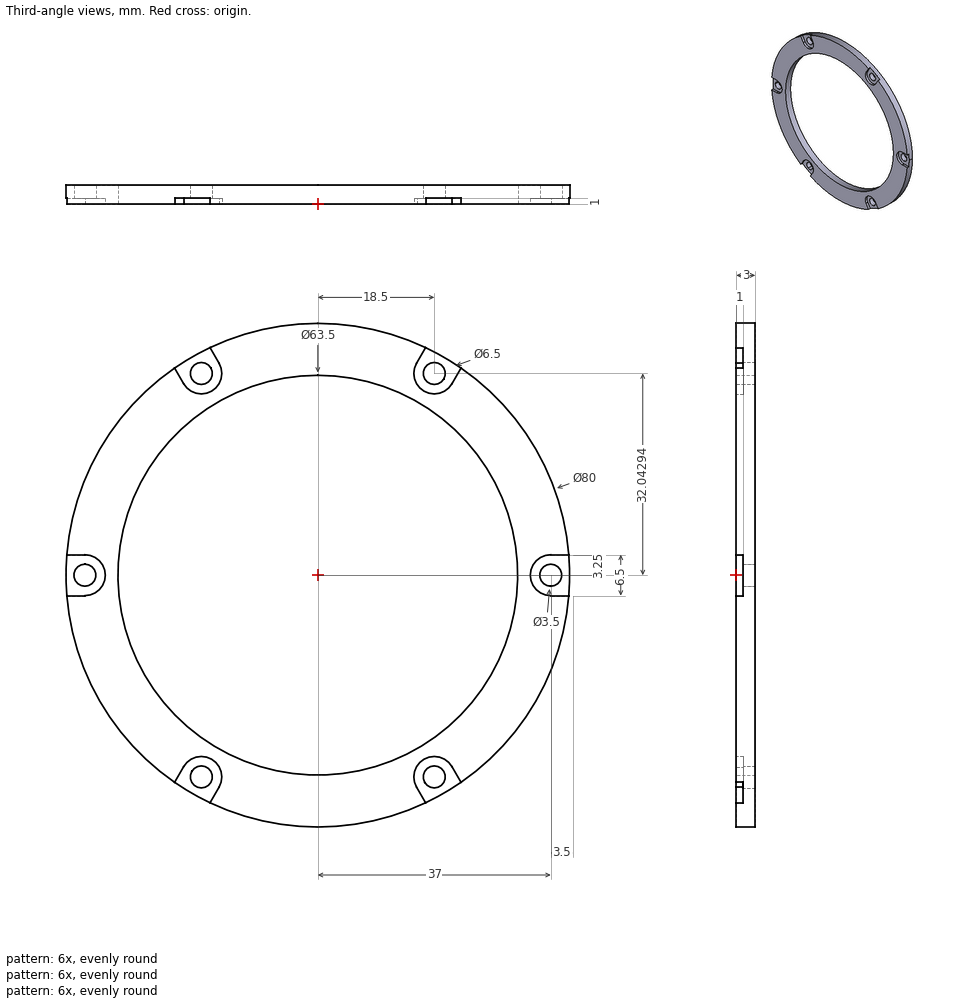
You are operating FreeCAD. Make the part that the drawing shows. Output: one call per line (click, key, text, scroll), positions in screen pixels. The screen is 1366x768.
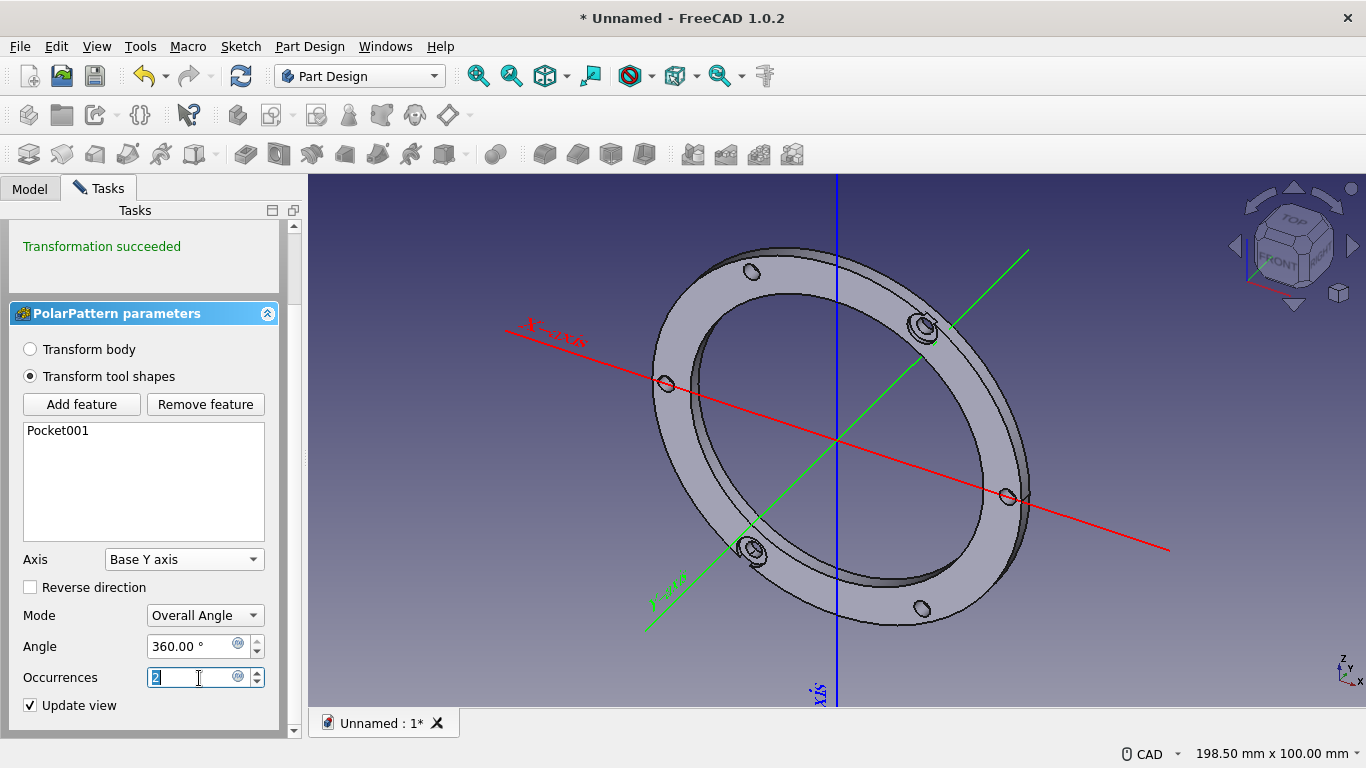
text(6)
key(Tab)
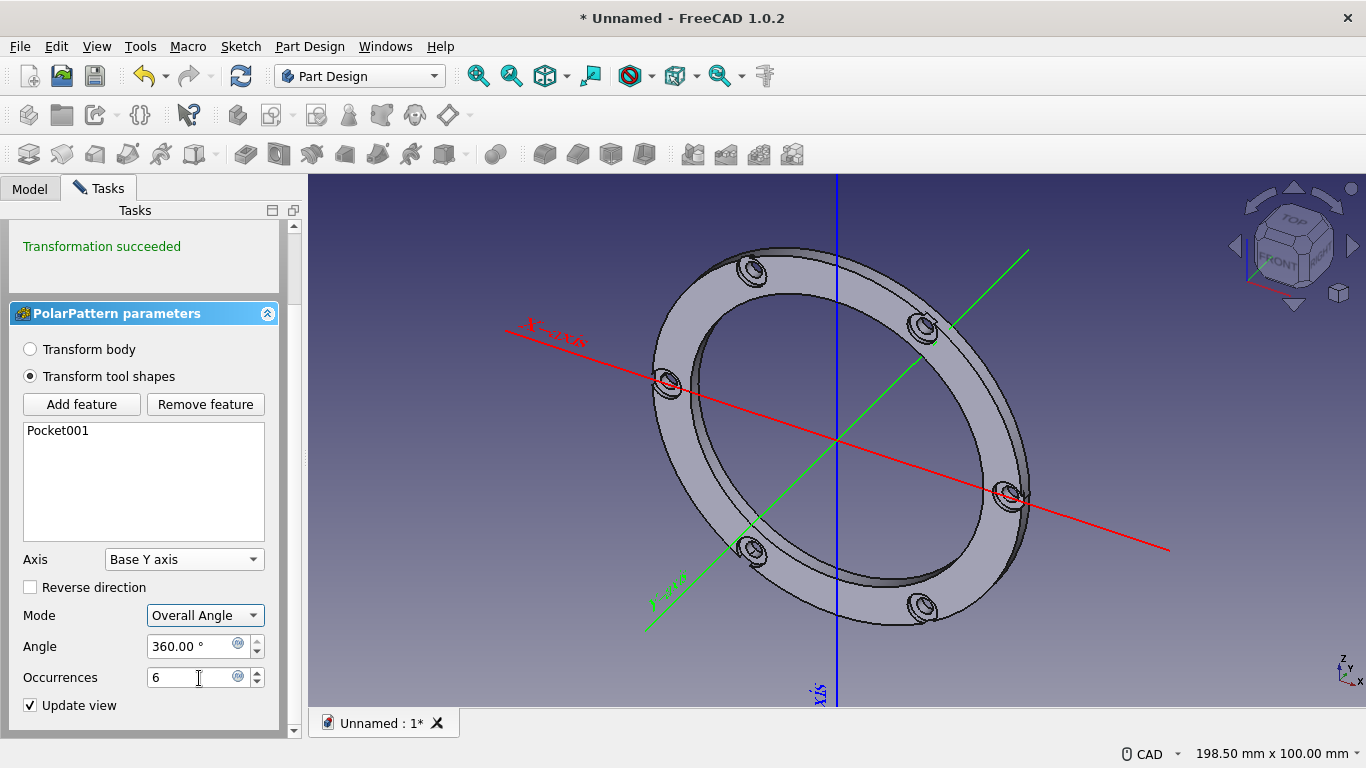
scroll(294, 479, up, 3)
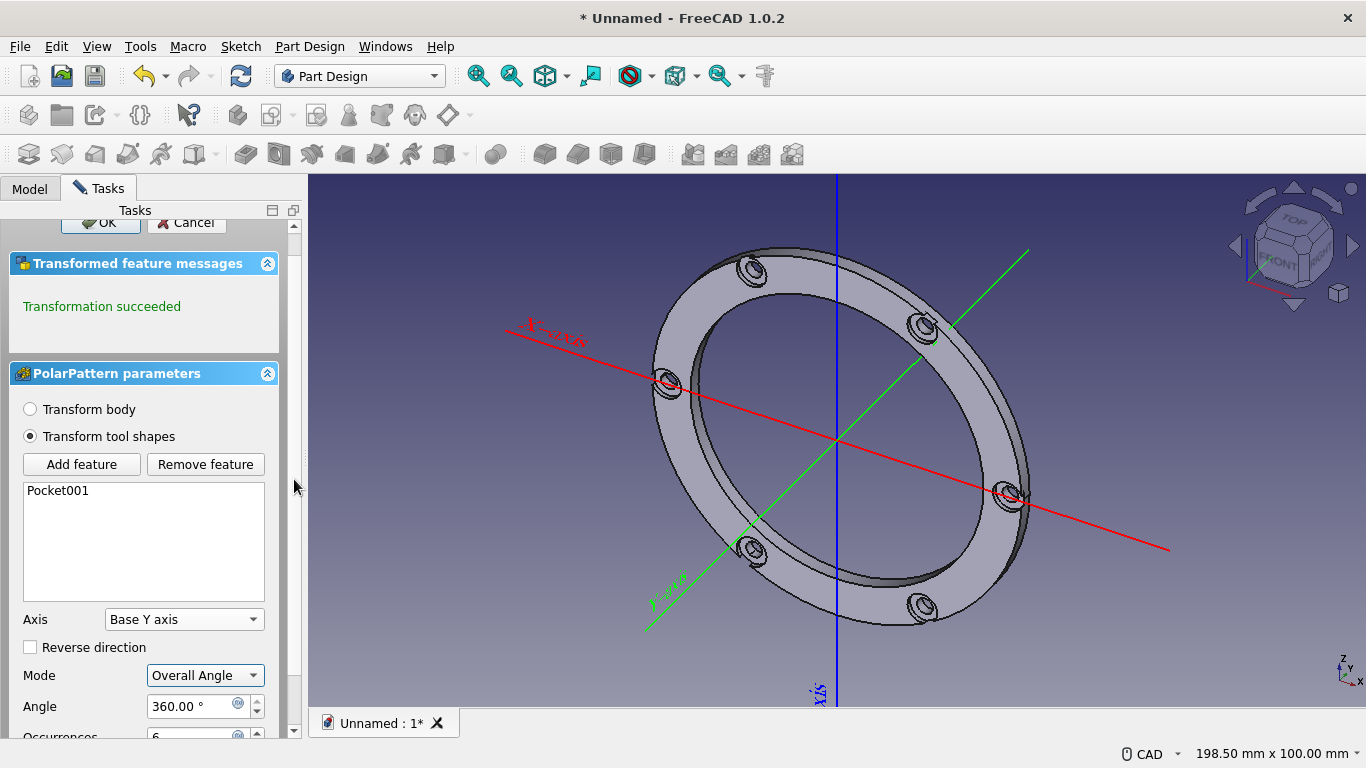
click(101, 249)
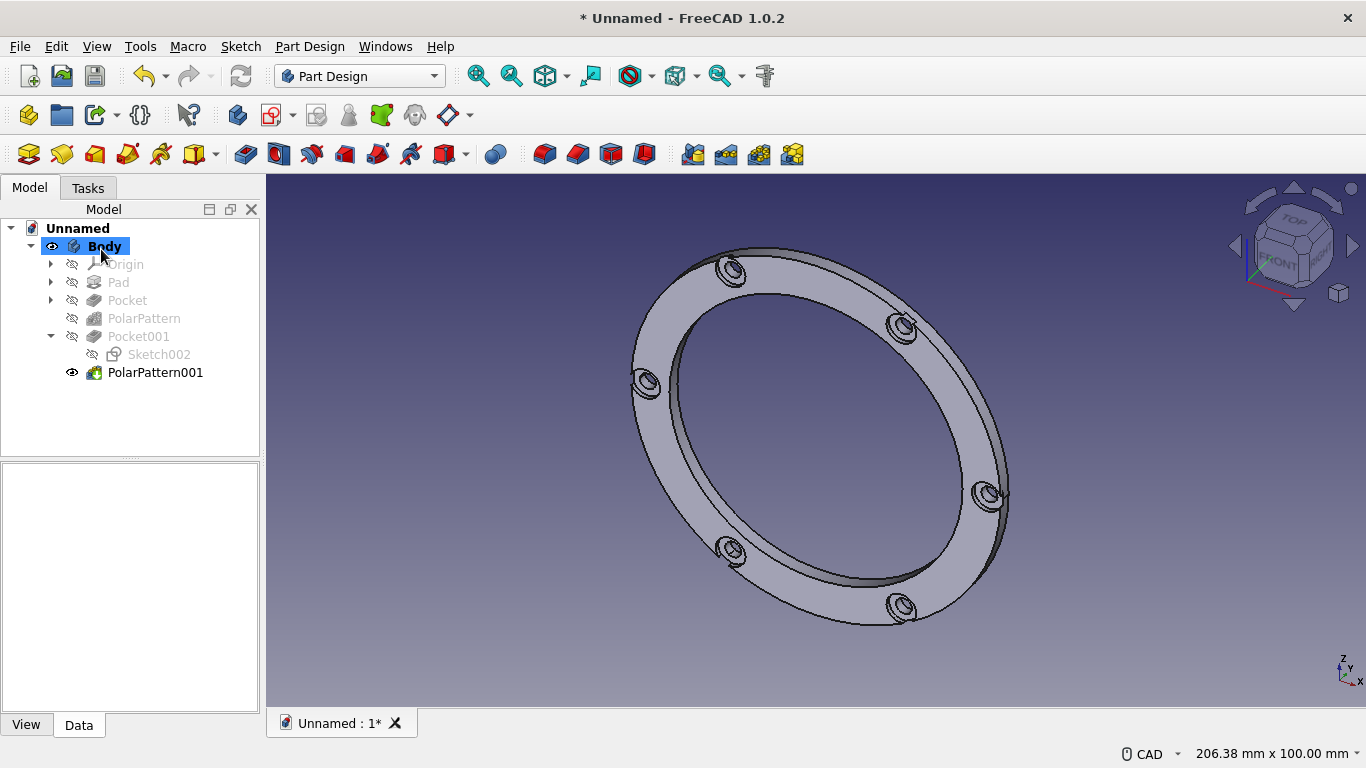
click(974, 542)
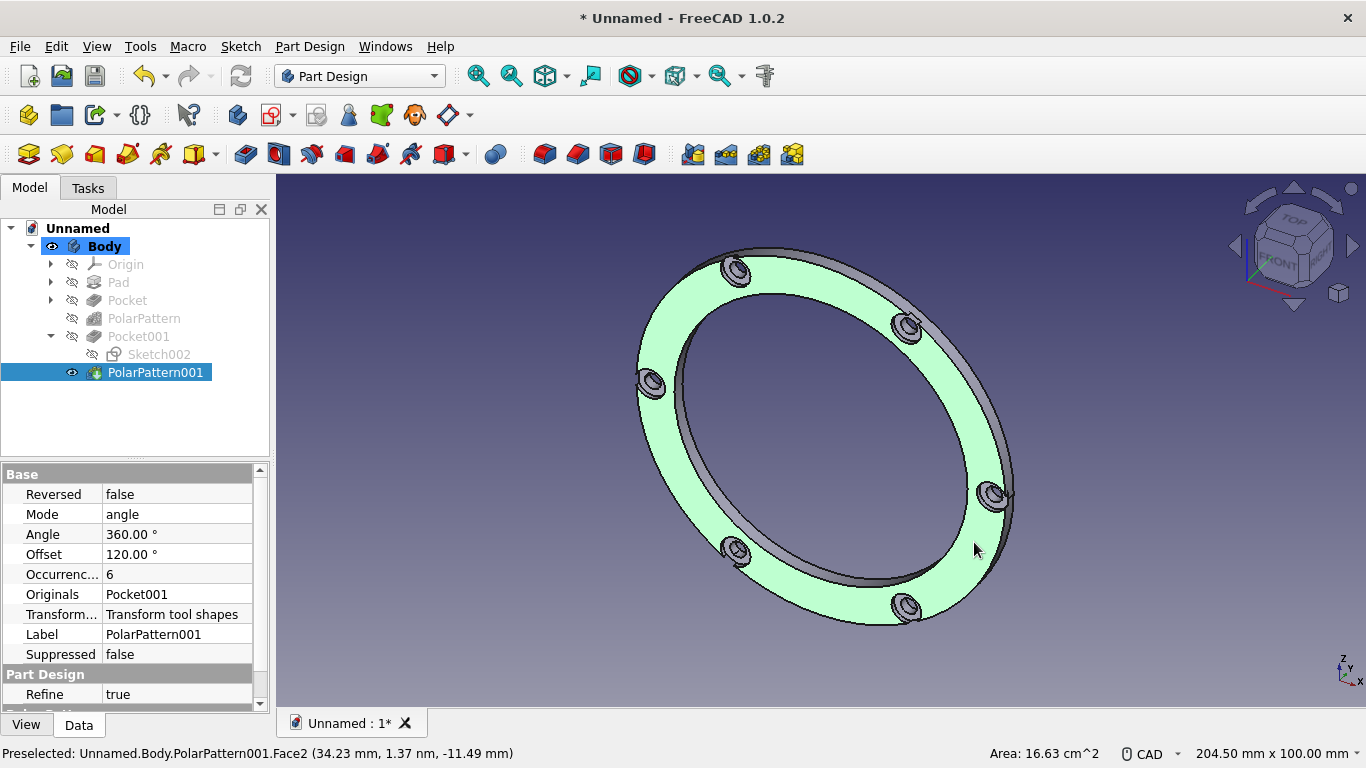
click(270, 116)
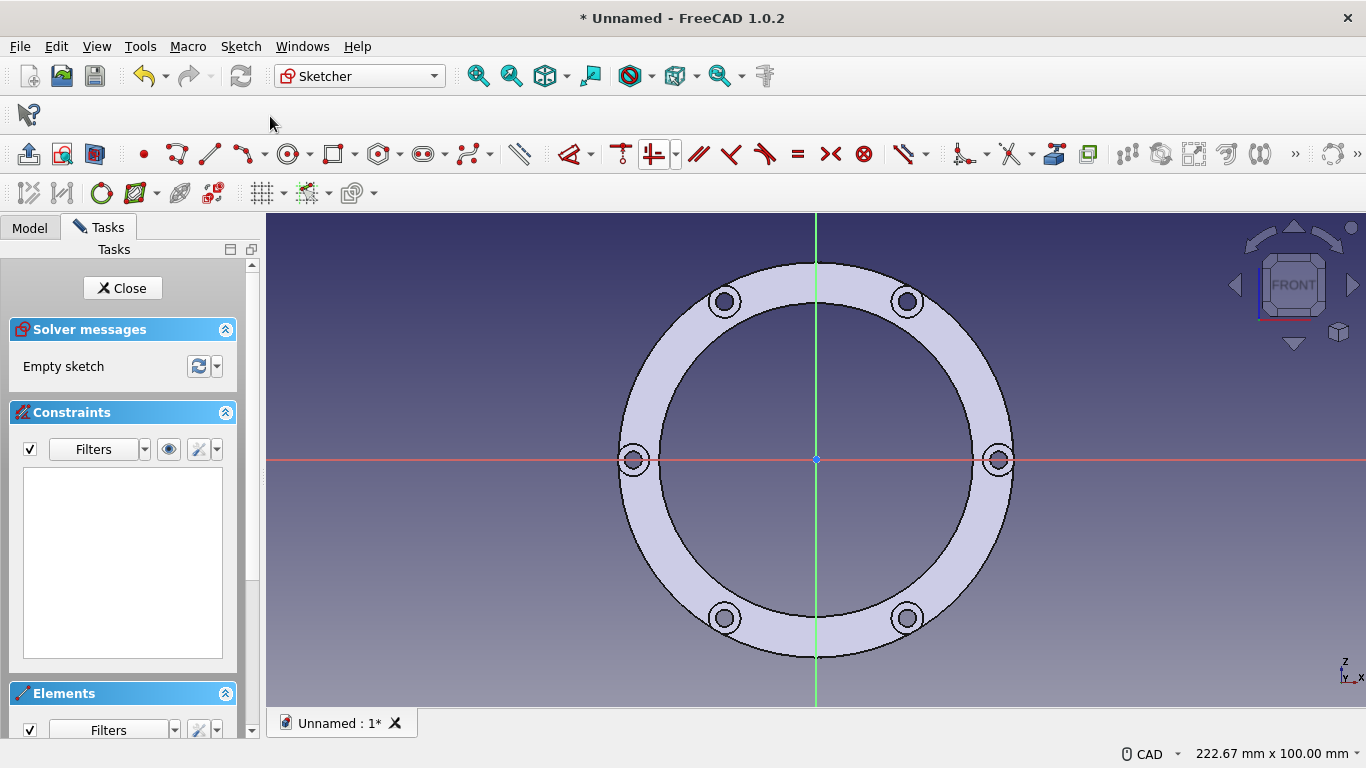
scroll(1040, 460, up, 11)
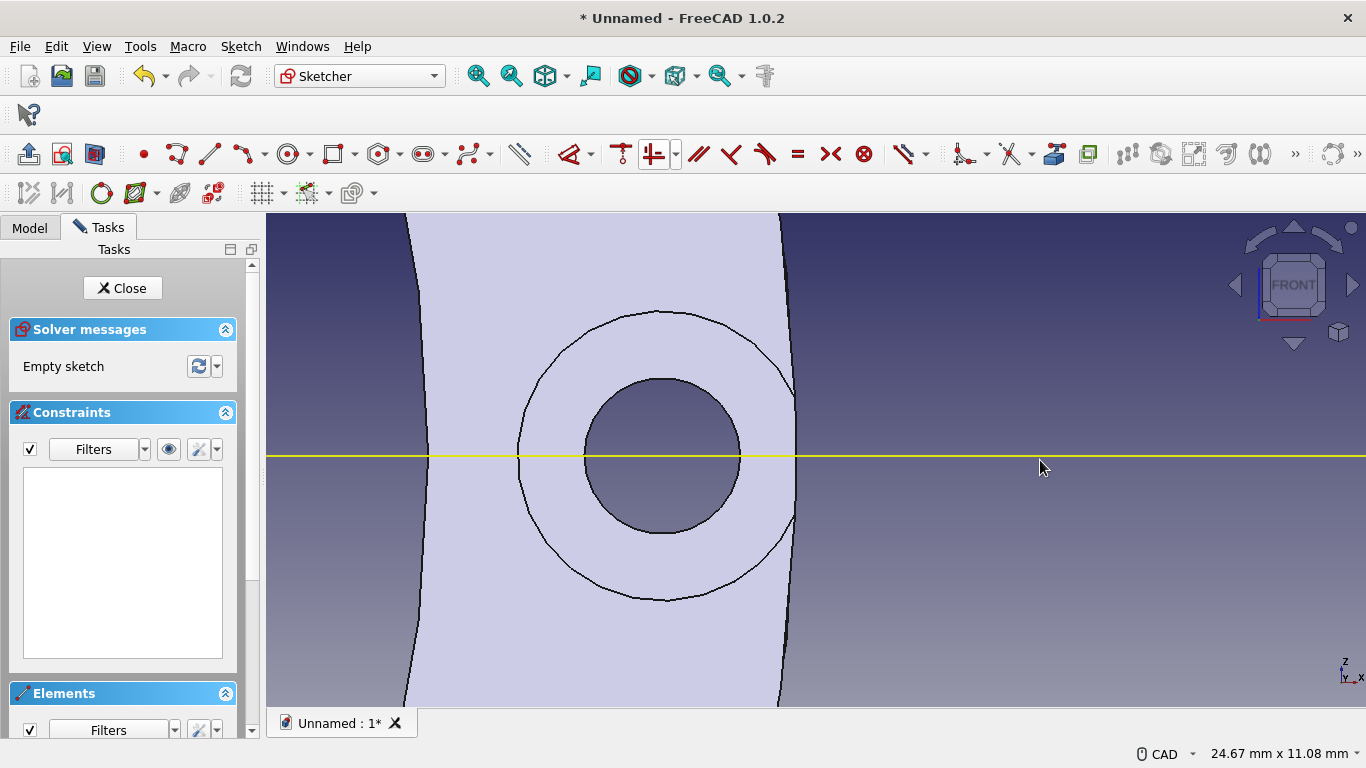
click(332, 154)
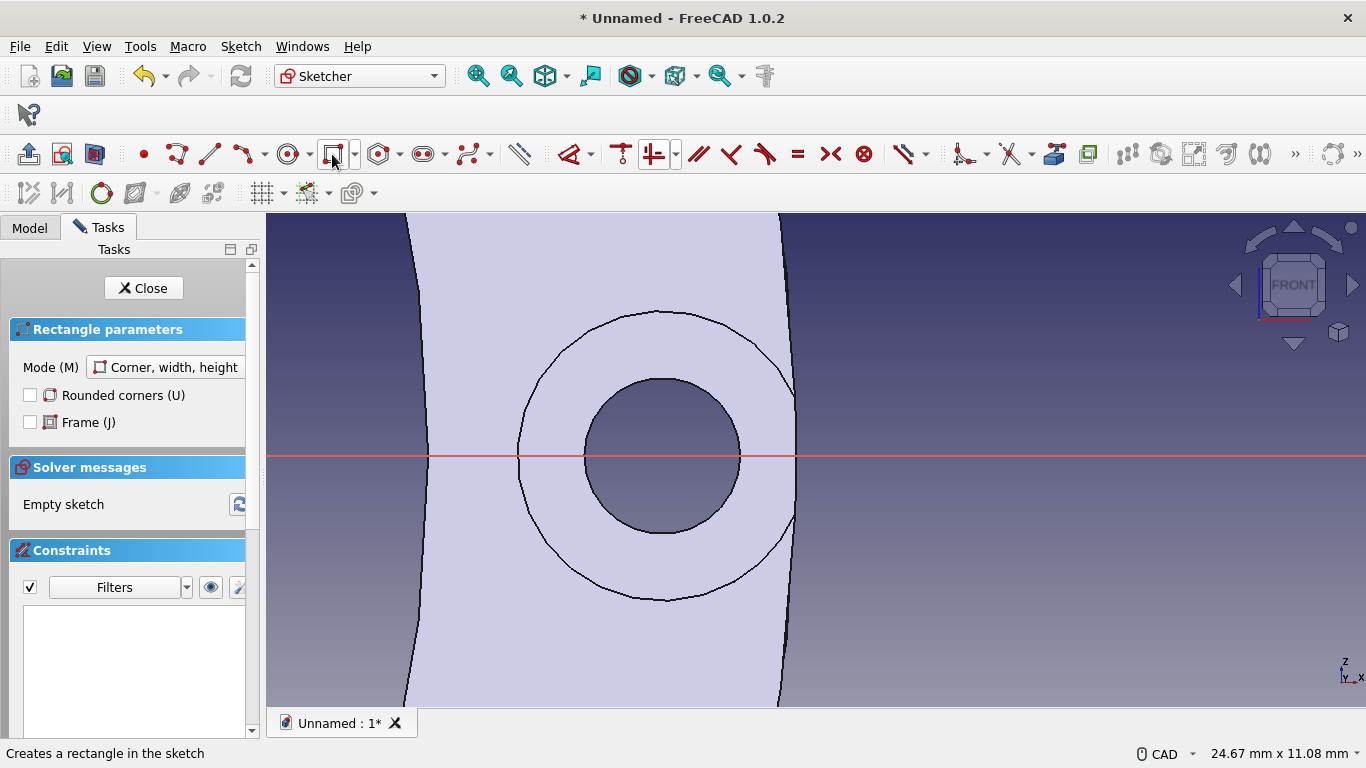
click(662, 311)
move(818, 601)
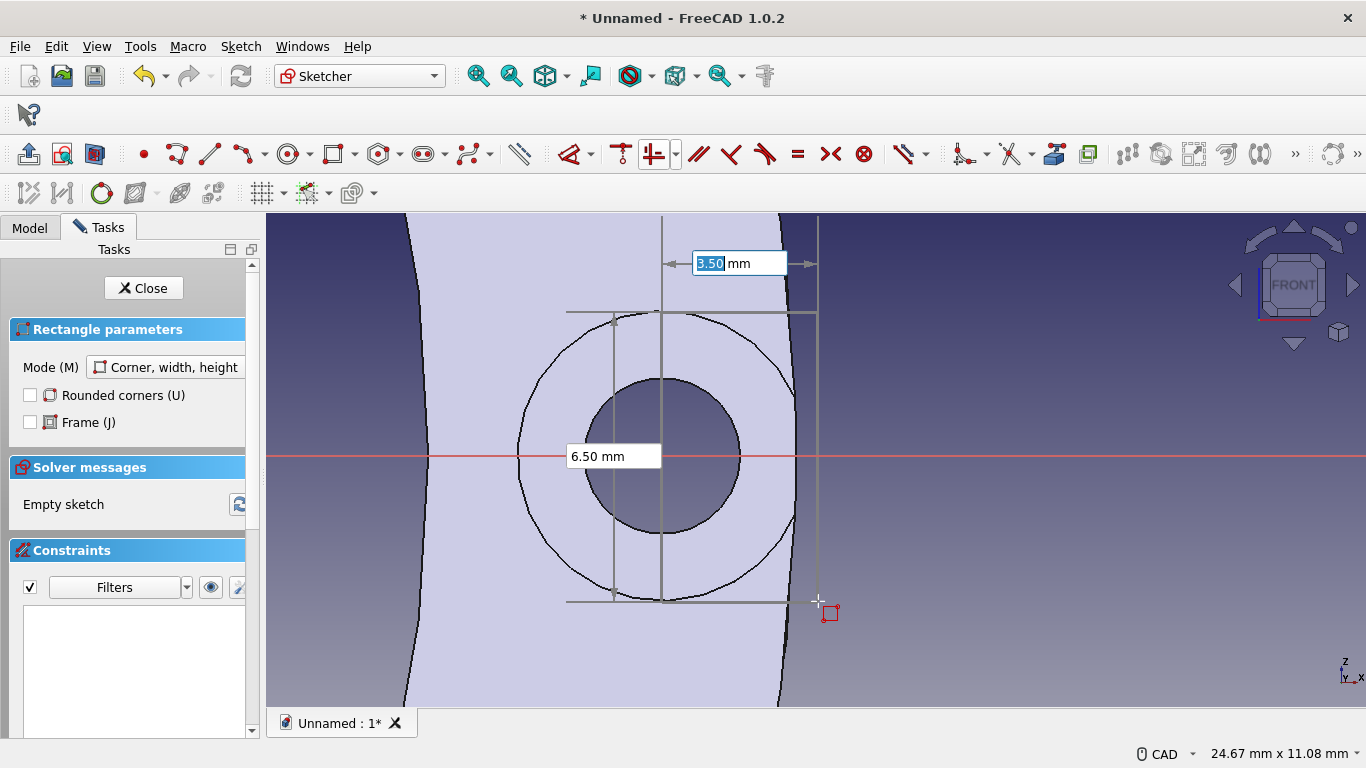
text(3.5)
key(Tab)
text(6.5)
key(Return)
key(Escape)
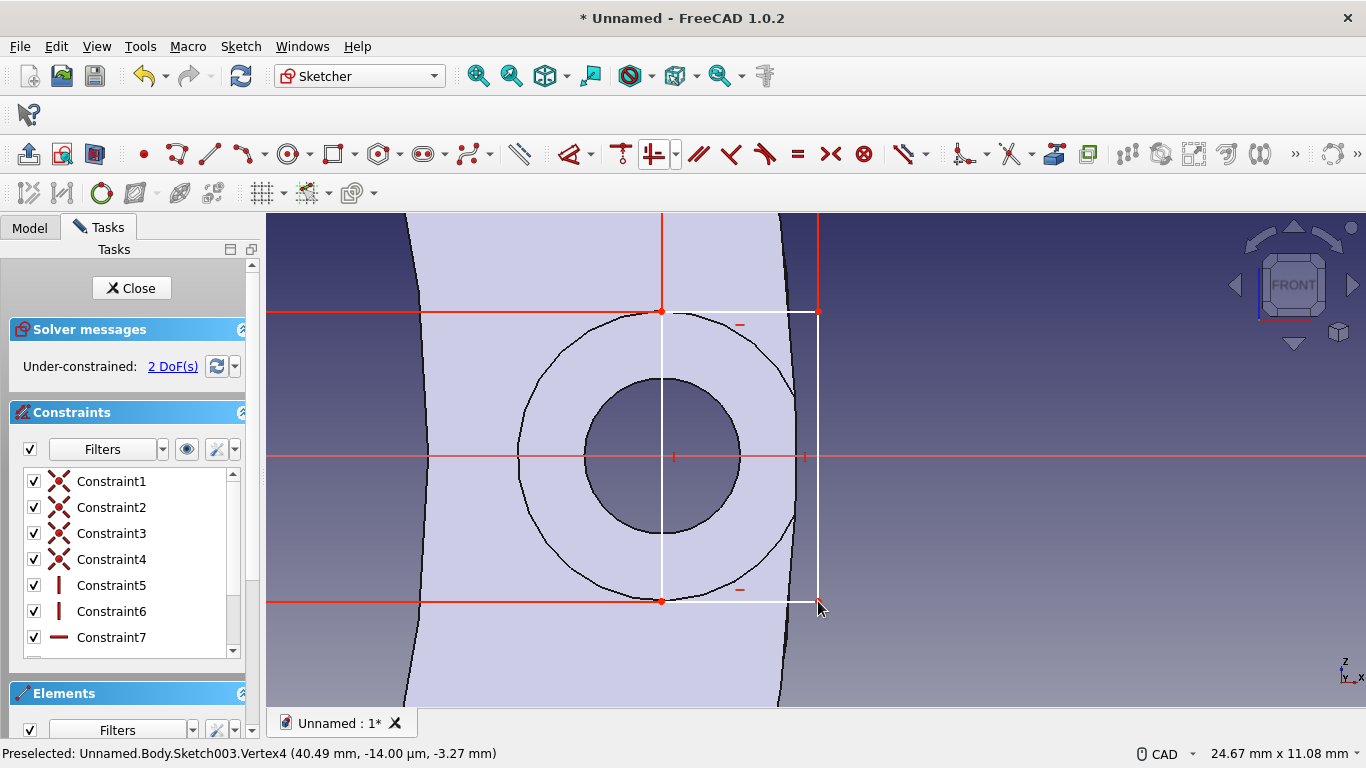
click(568, 154)